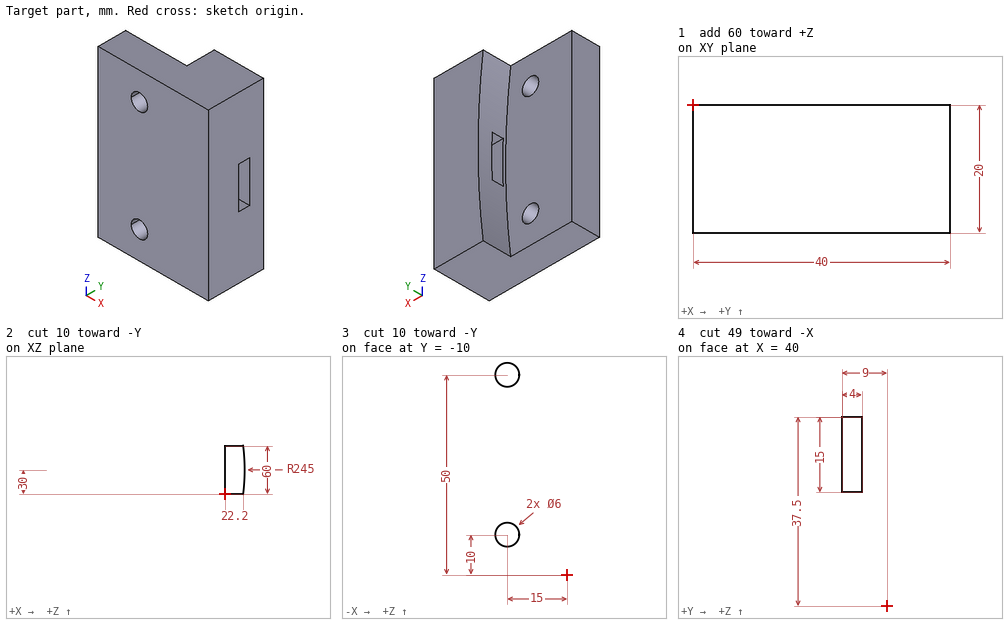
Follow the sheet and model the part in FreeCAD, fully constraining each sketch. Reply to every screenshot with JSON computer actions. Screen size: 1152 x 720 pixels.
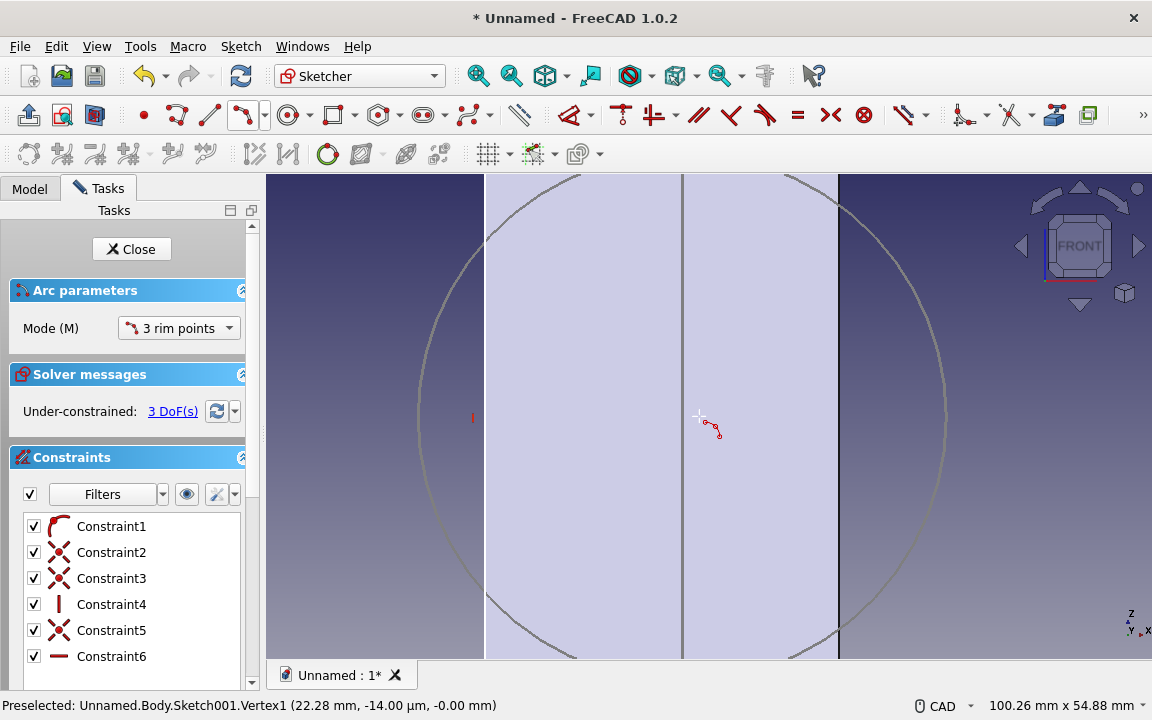
{"action": "left_click", "coordinate": [698, 416]}
{"action": "key", "text": "Escape"}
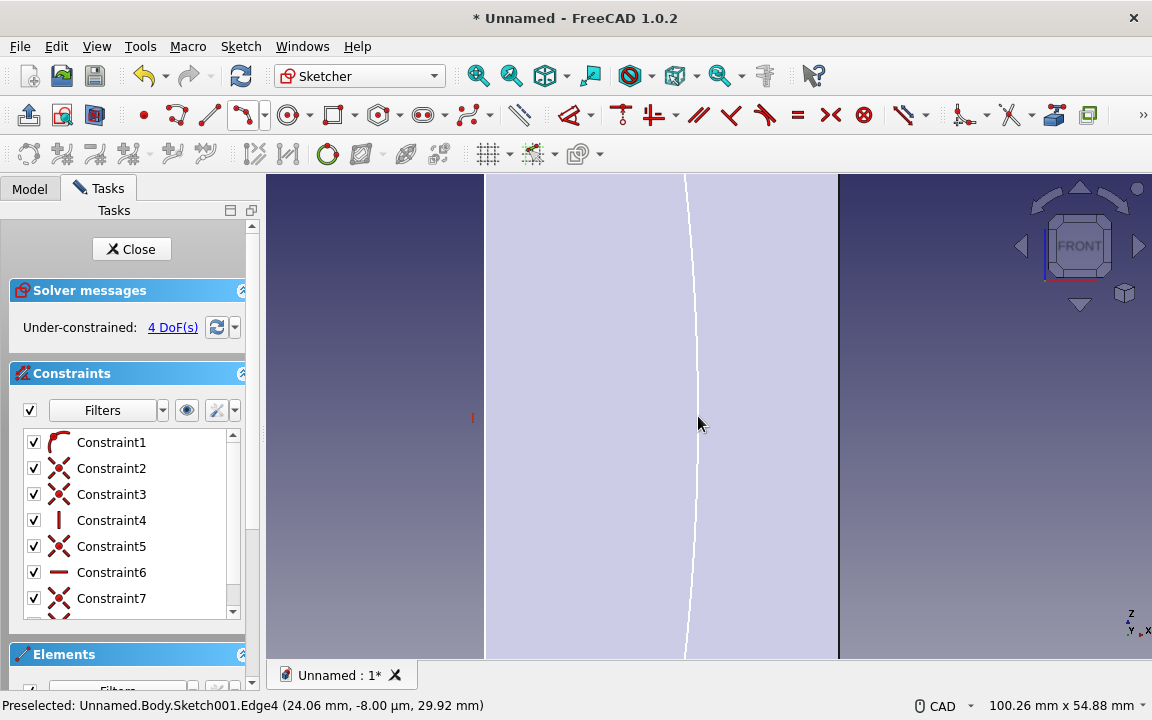
{"action": "left_click", "coordinate": [568, 116]}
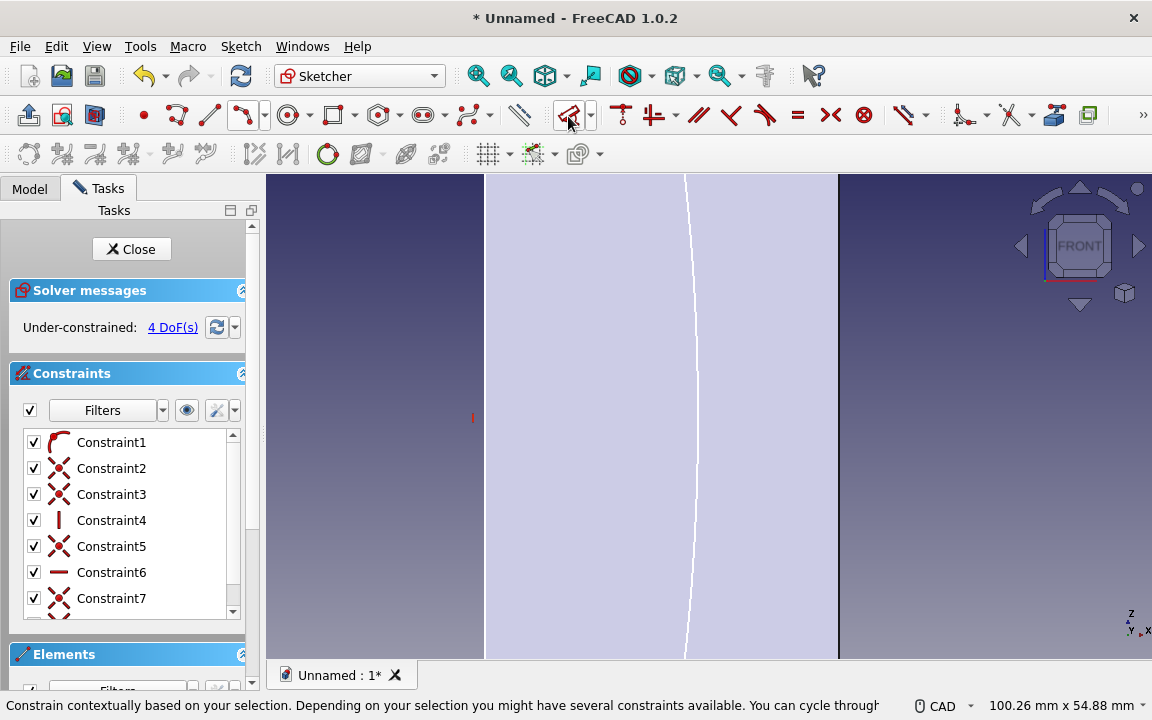
{"action": "left_click", "coordinate": [695, 523]}
{"action": "left_click", "coordinate": [727, 525]}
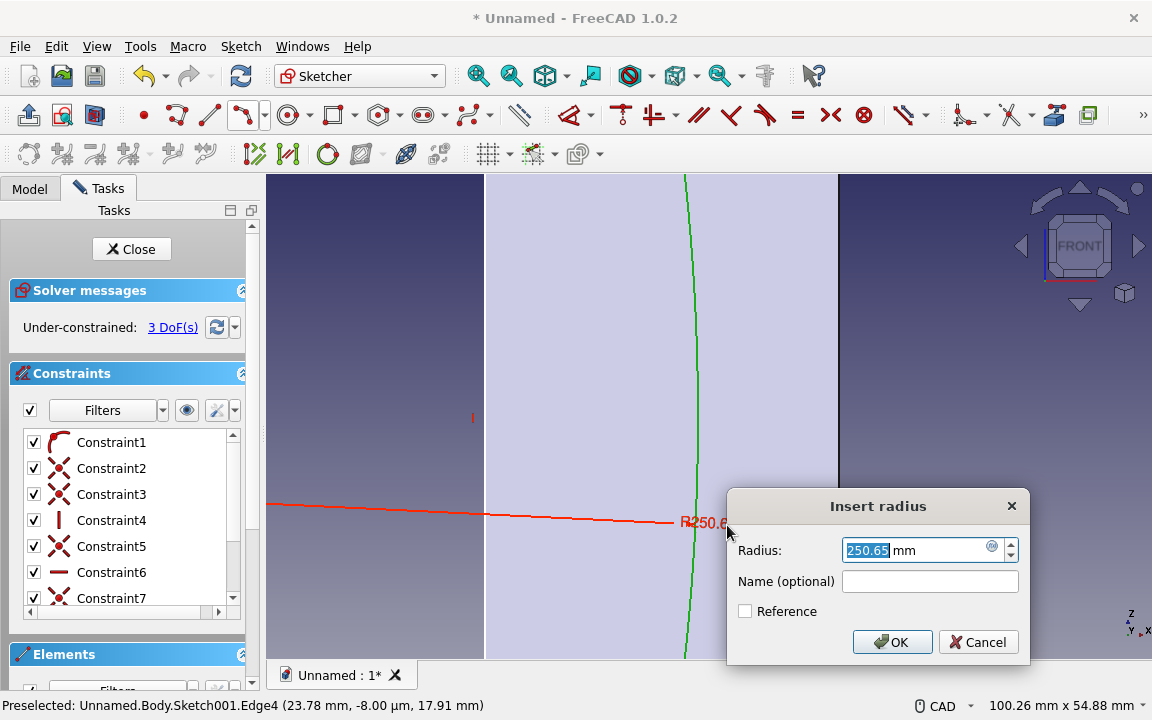
{"action": "type", "text": "245"}
{"action": "key", "text": "Return"}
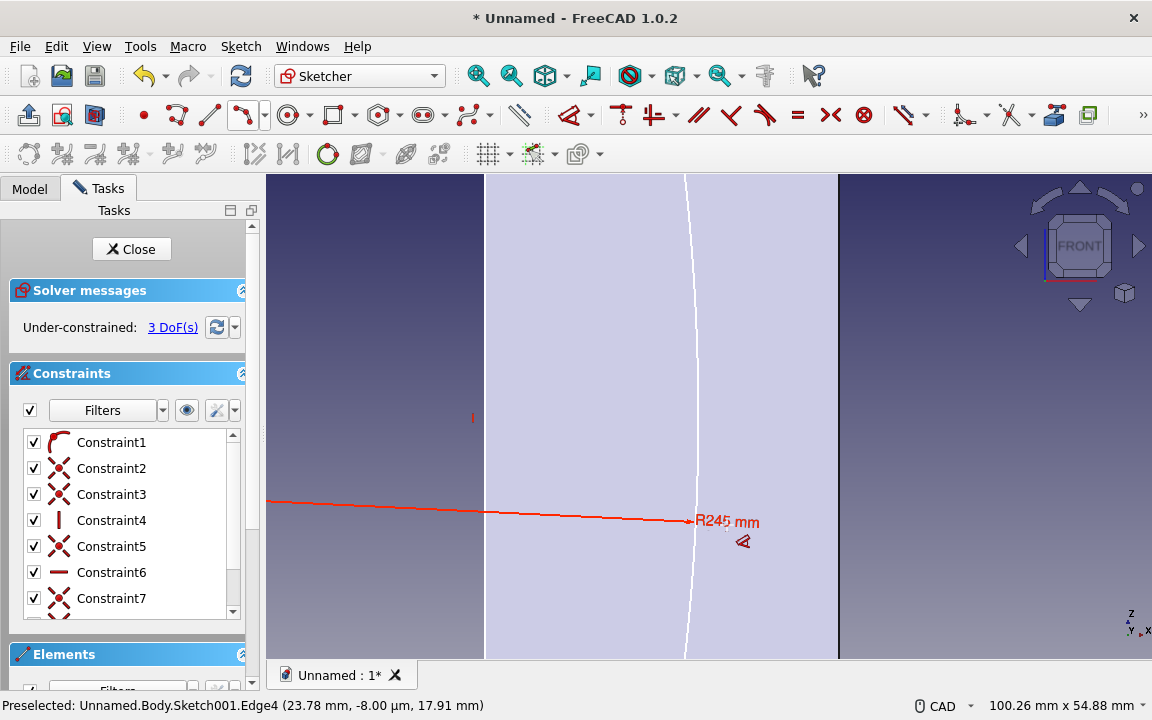
{"action": "left_click", "coordinate": [485, 523]}
{"action": "left_click", "coordinate": [451, 416]}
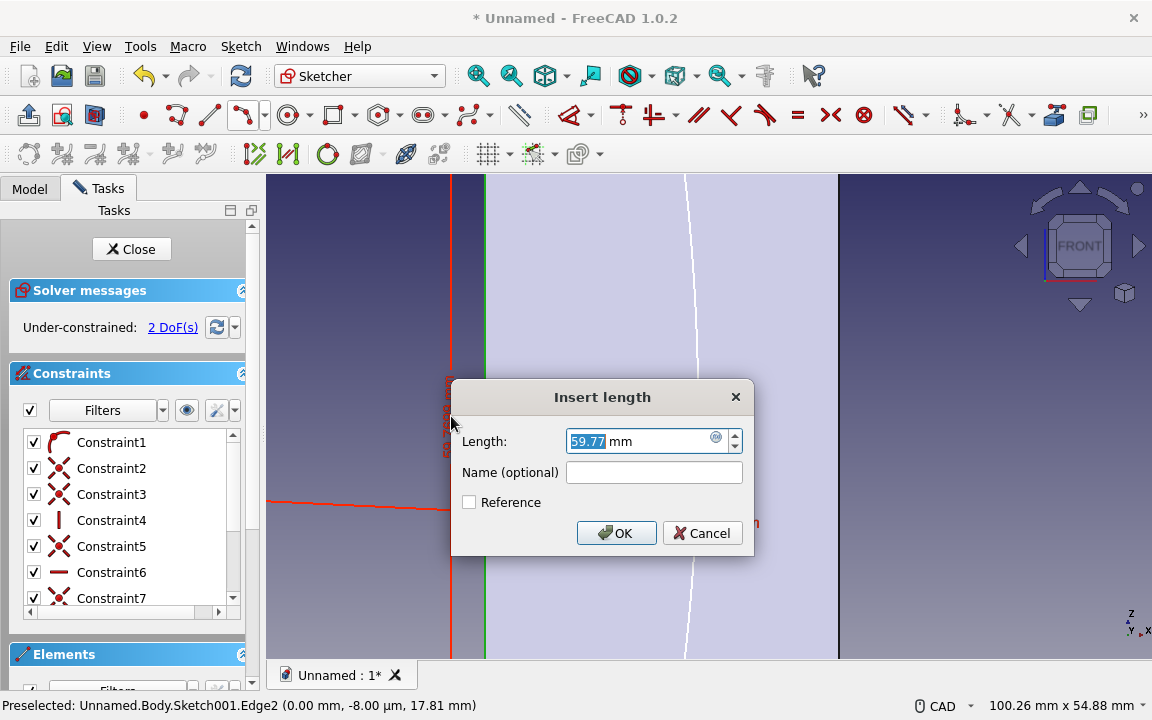
{"action": "type", "text": "60"}
{"action": "key", "text": "Return"}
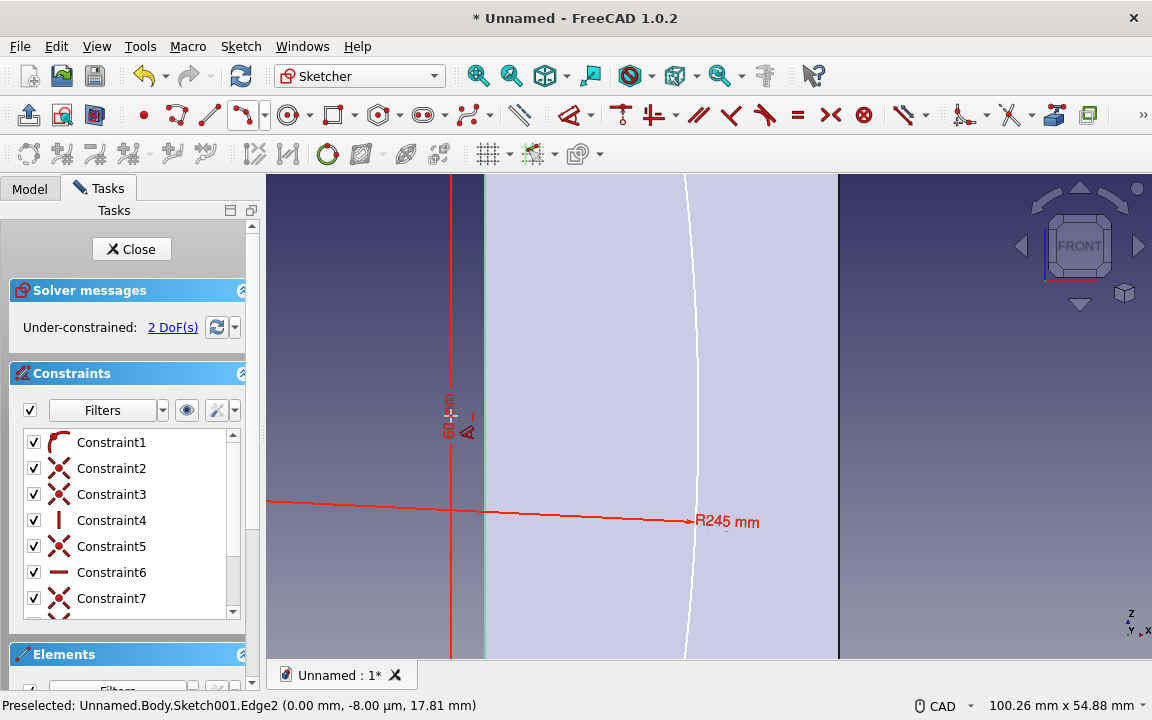
{"action": "scroll", "coordinate": [700, 417], "scroll_direction": "down", "scroll_amount": 3}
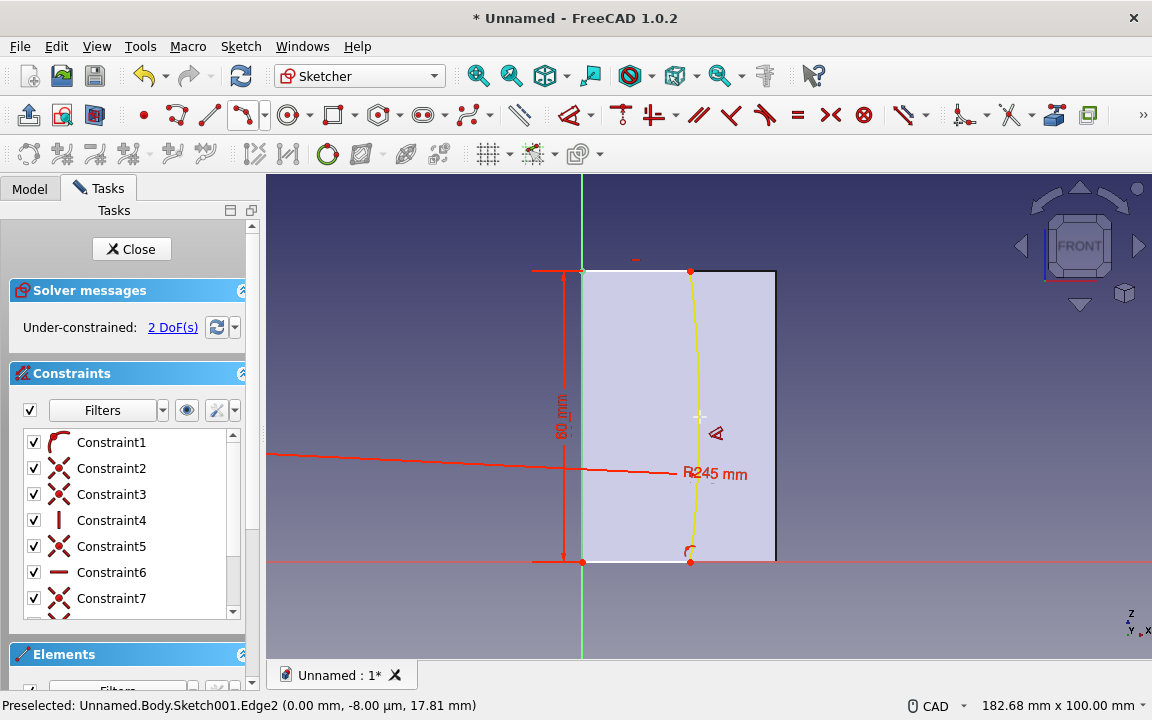
{"action": "scroll", "coordinate": [987, 416], "scroll_direction": "down", "scroll_amount": 4}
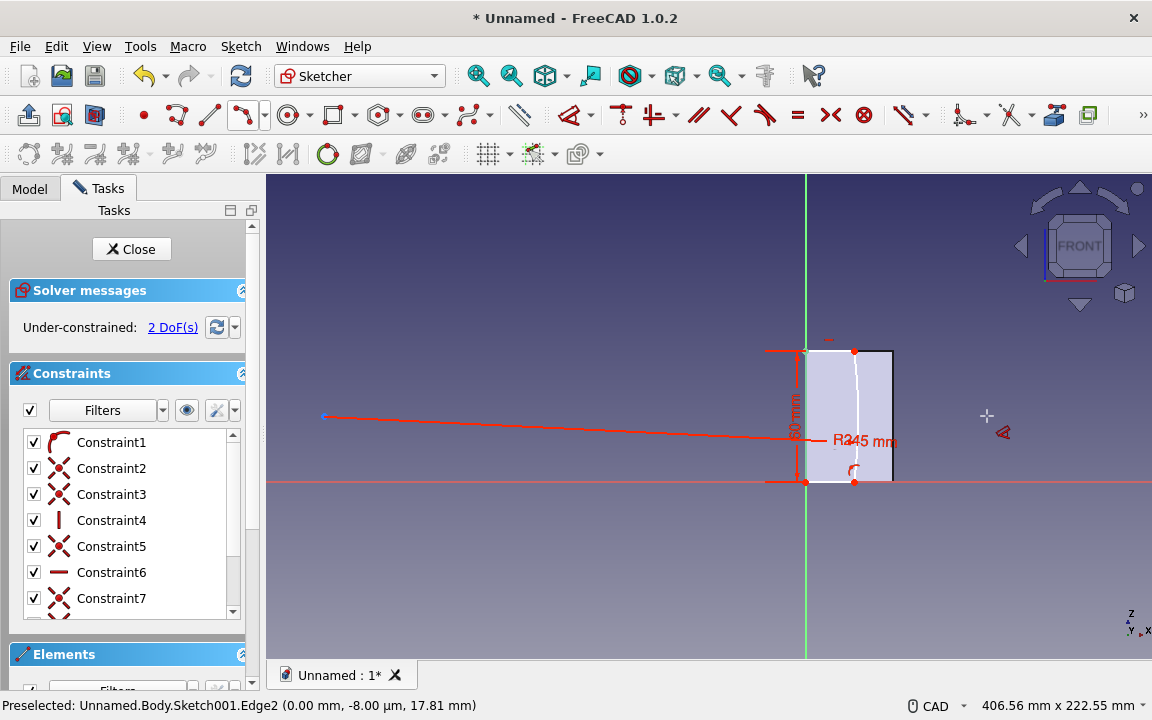
{"action": "left_click", "coordinate": [324, 417]}
{"action": "left_click", "coordinate": [840, 464]}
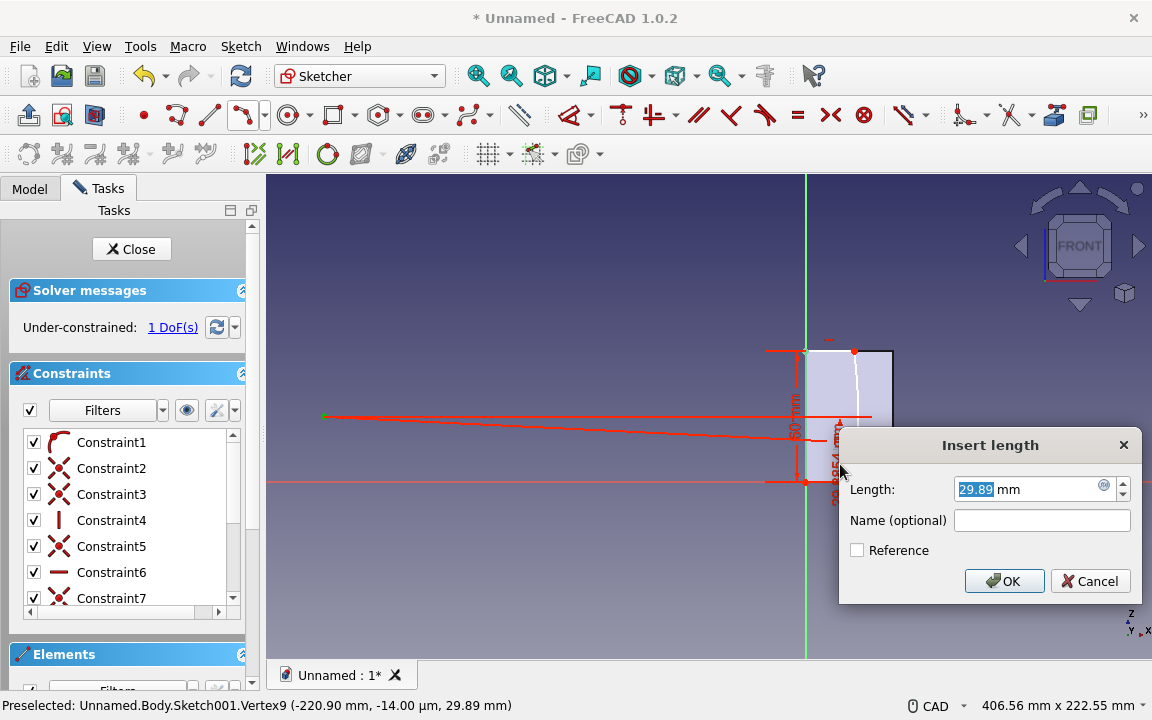
{"action": "type", "text": "30"}
{"action": "key", "text": "Return"}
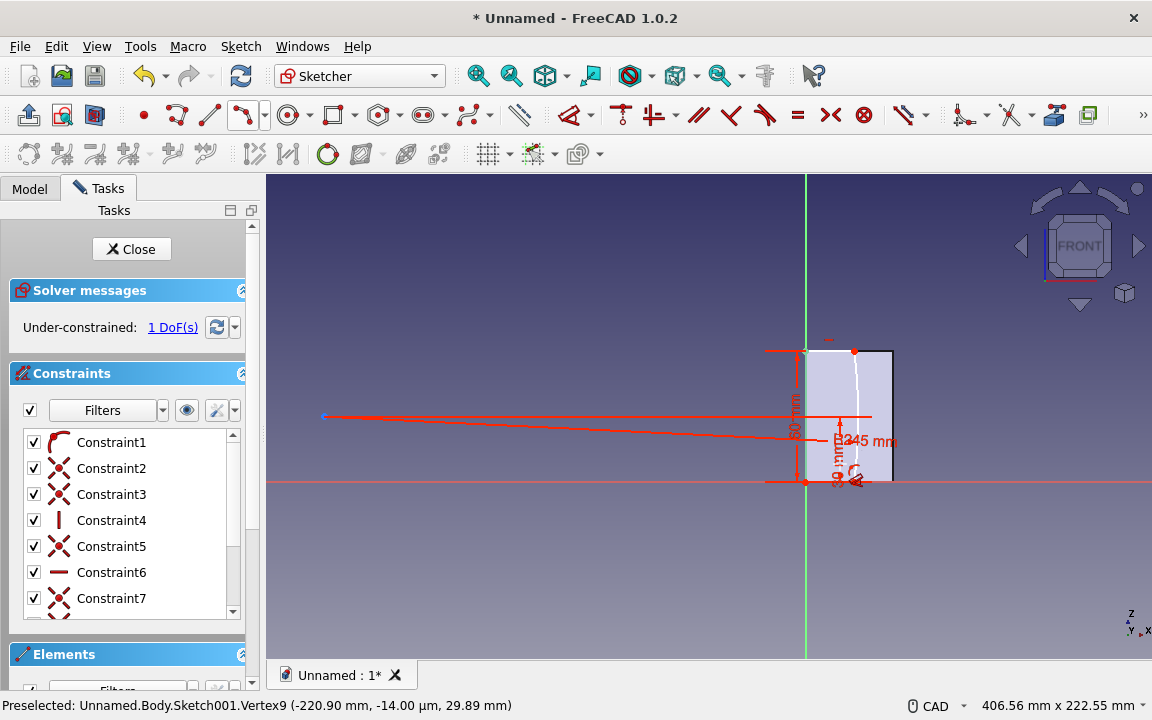
{"action": "left_click", "coordinate": [840, 482]}
{"action": "left_click", "coordinate": [830, 516]}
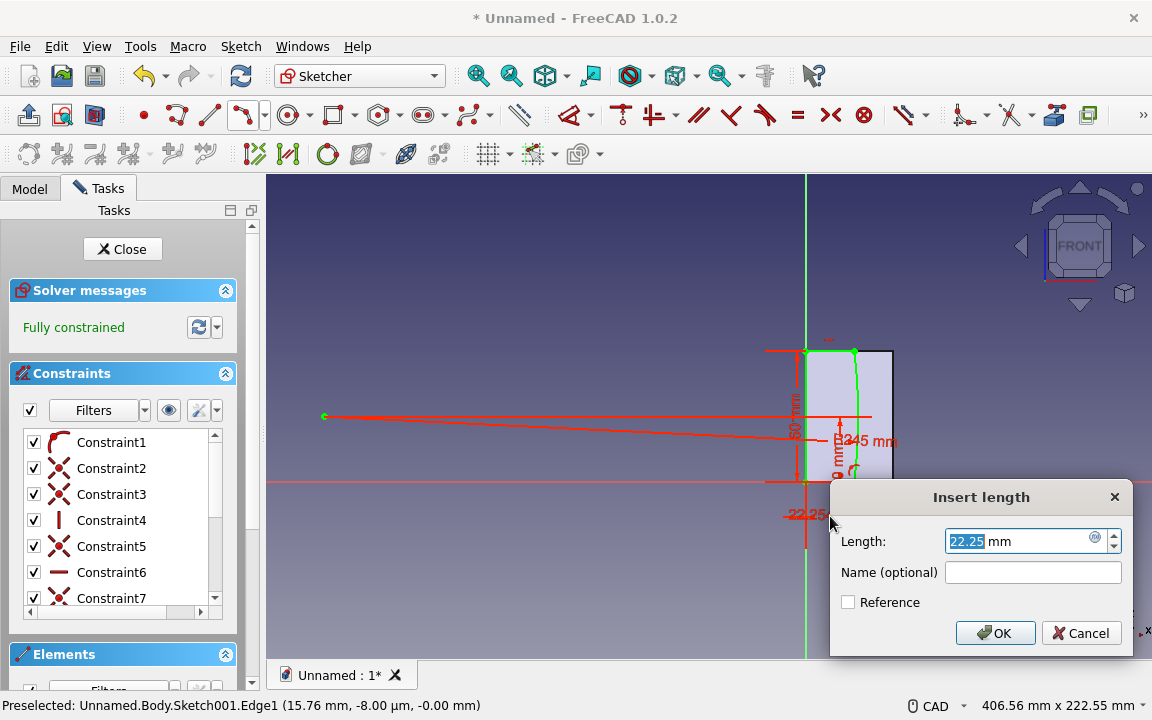
{"action": "type", "text": "22.2"}
{"action": "key", "text": "Return"}
{"action": "key", "text": "Escape"}